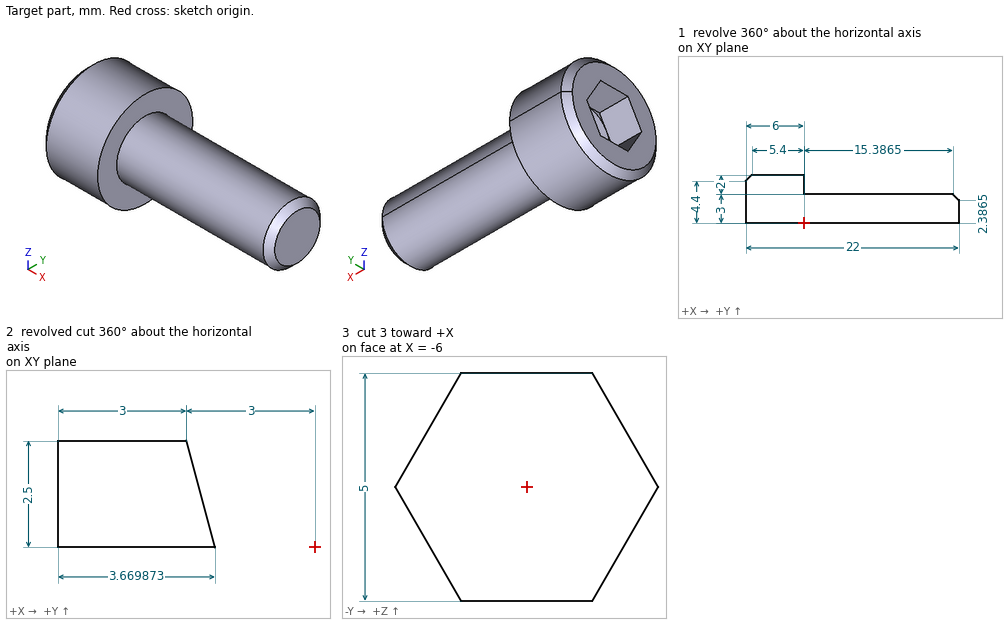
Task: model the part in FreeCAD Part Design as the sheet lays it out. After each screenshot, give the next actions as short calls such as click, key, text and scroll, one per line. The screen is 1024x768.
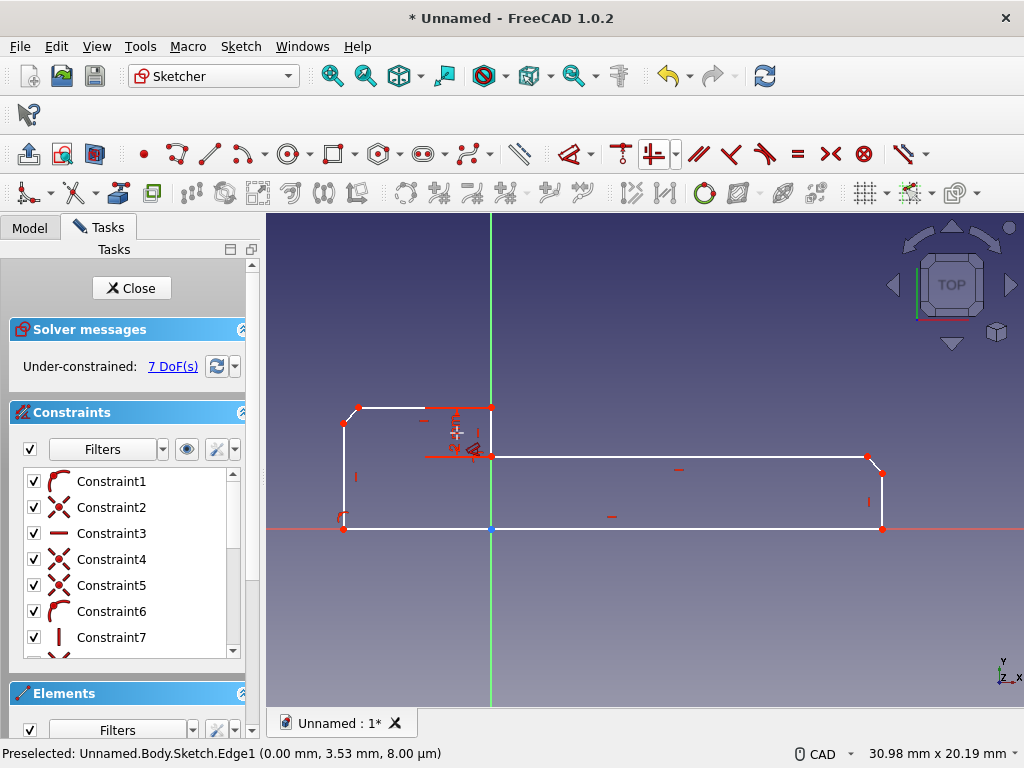
click(505, 529)
click(601, 563)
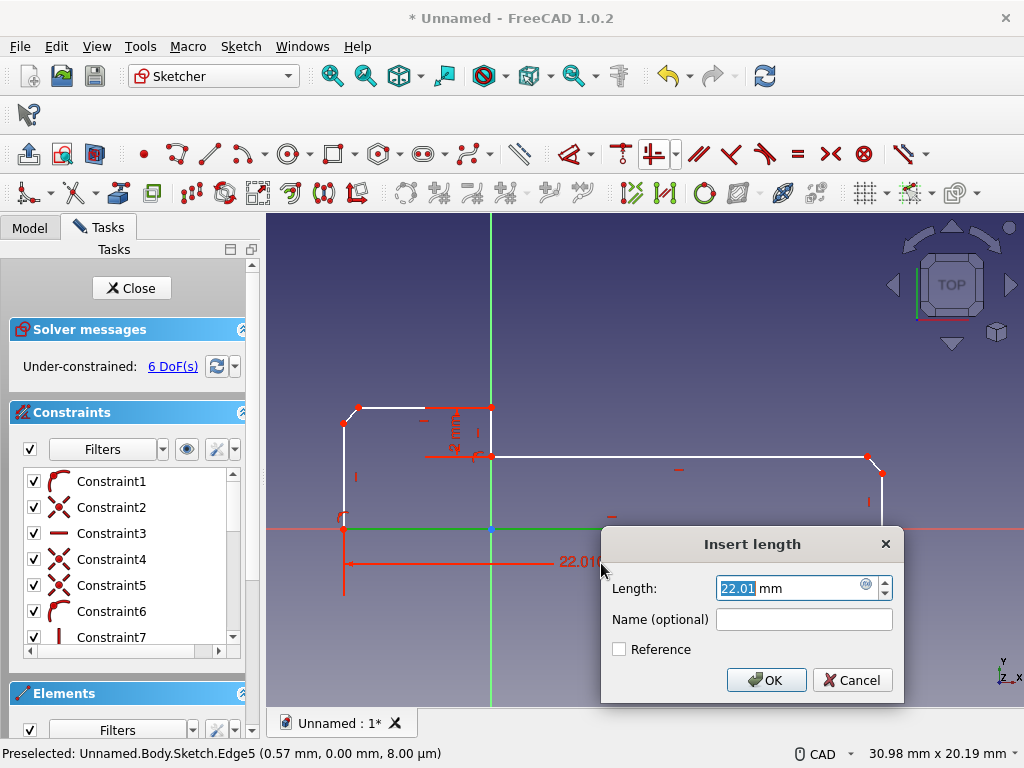
text(22)
key(Return)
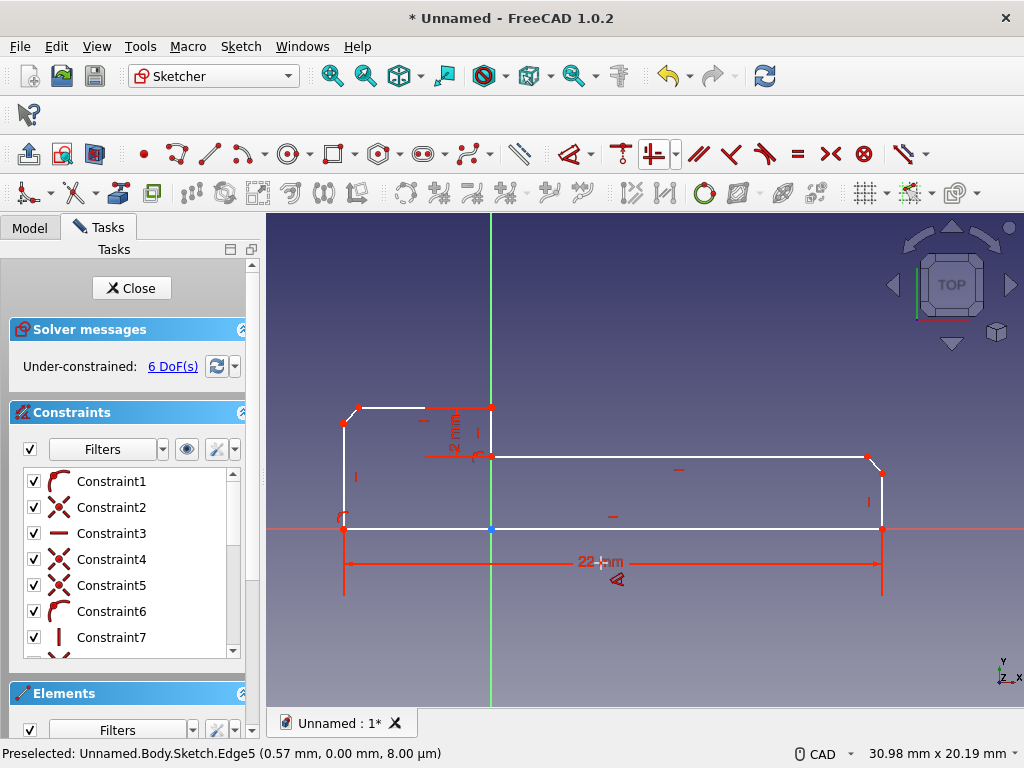
click(491, 457)
click(457, 493)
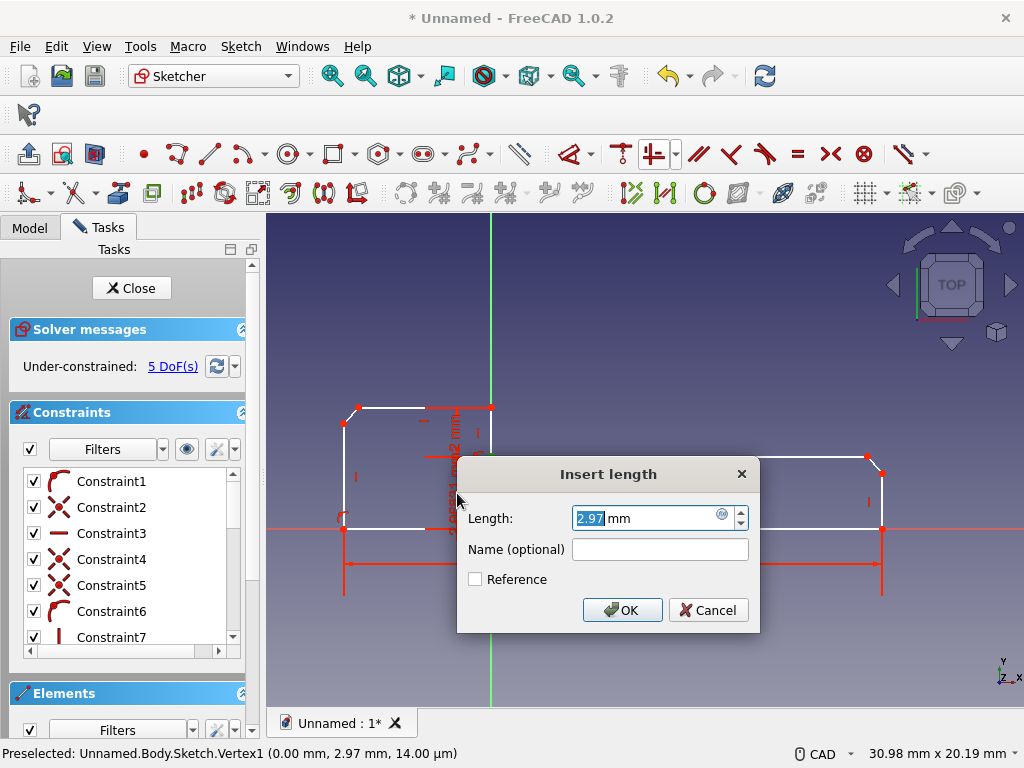
text(3)
key(Return)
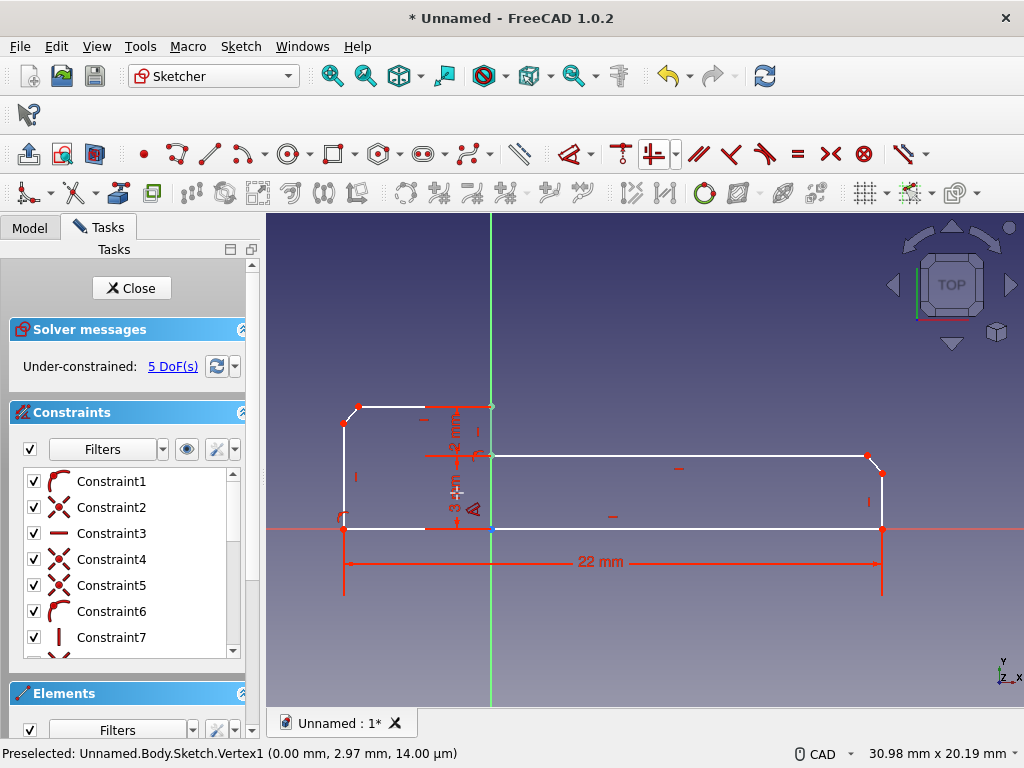
click(344, 424)
click(418, 563)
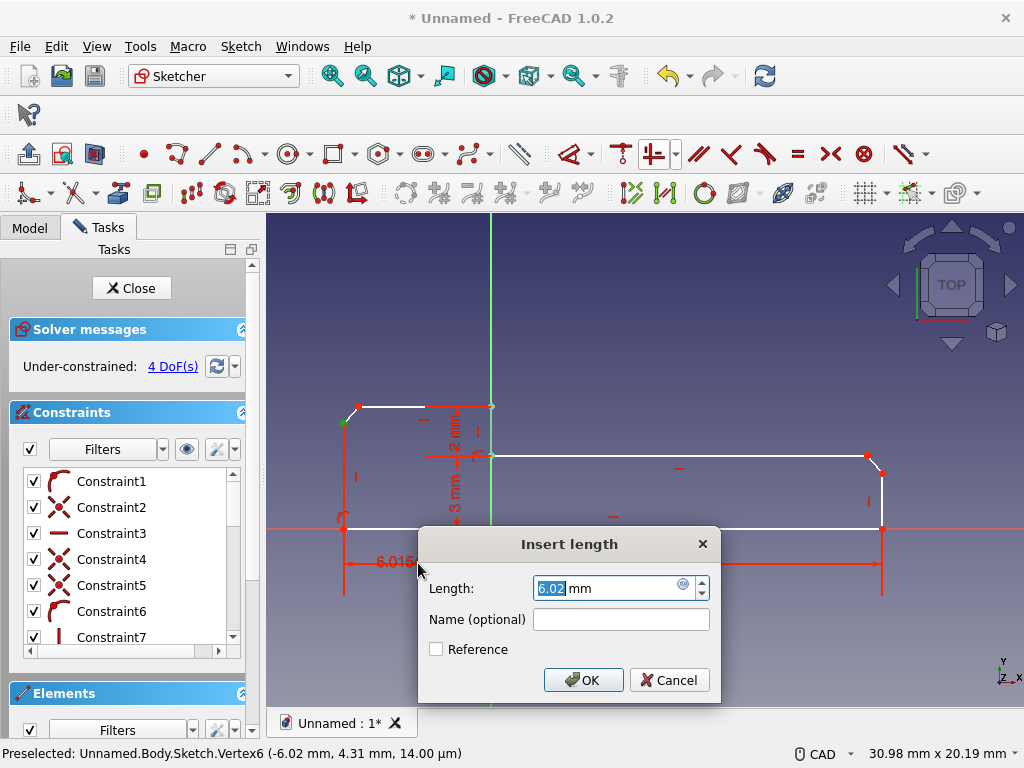
text(6)
key(Return)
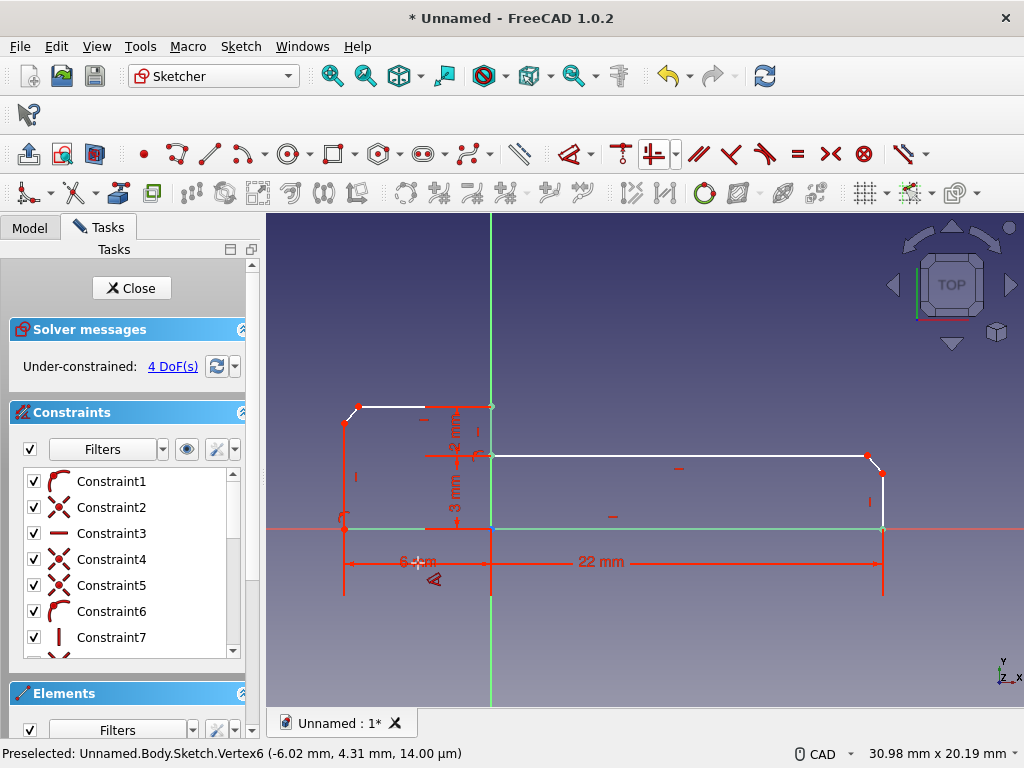
click(451, 407)
click(425, 373)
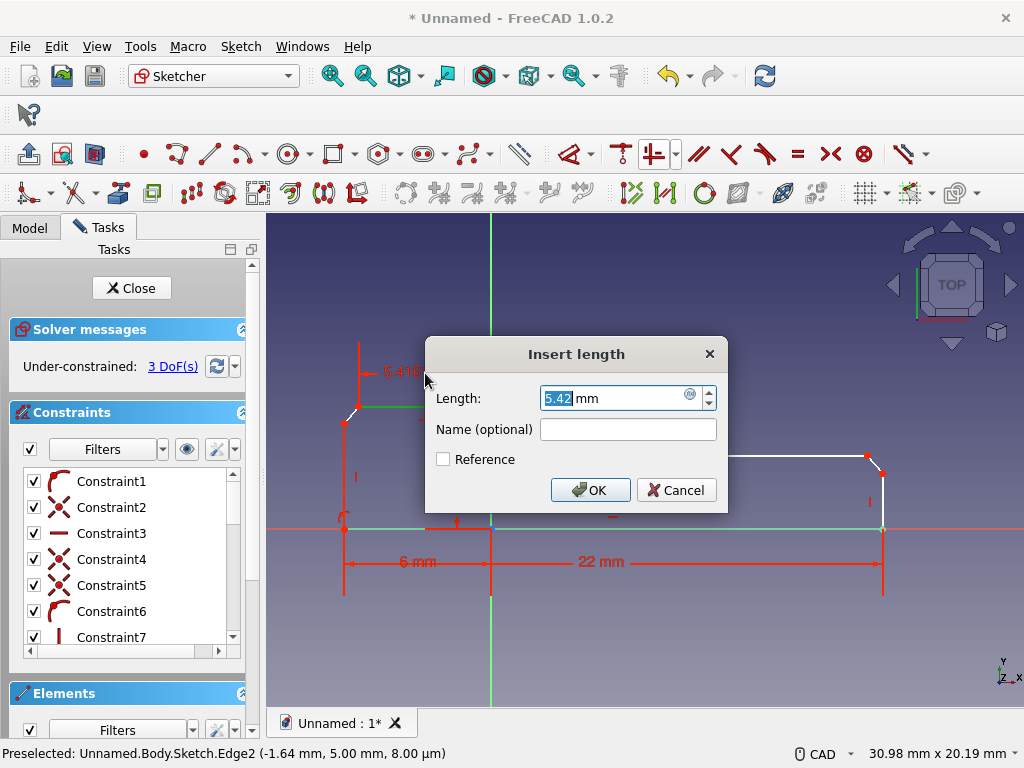
text(5.4)
key(Return)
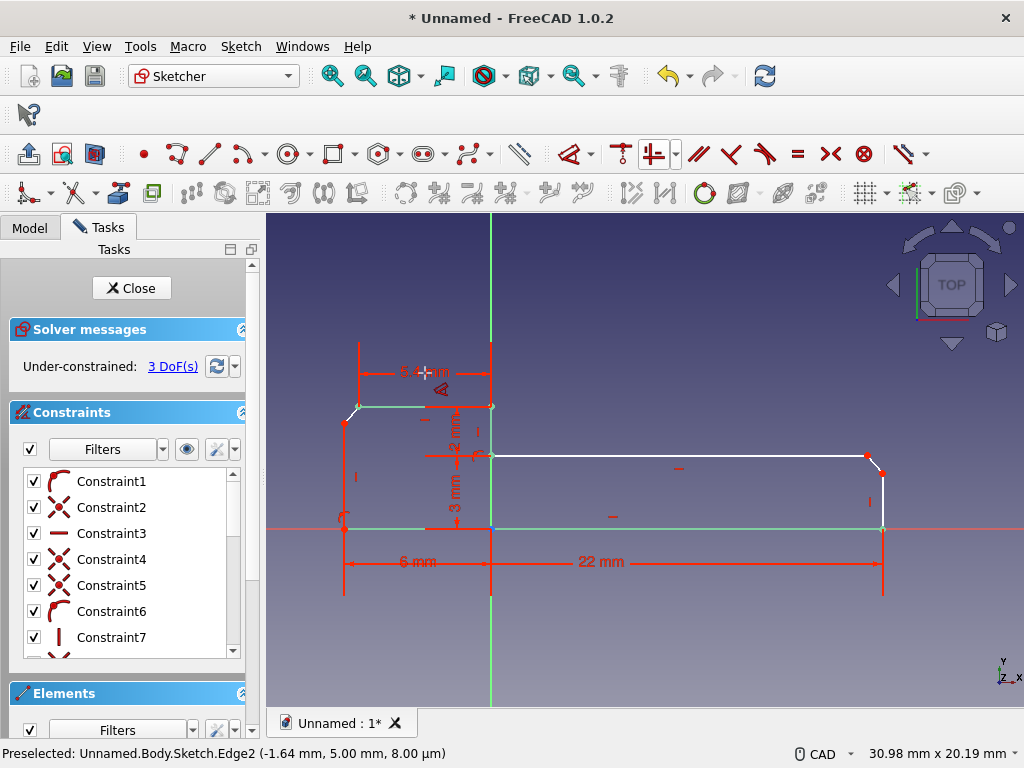
click(344, 456)
click(310, 477)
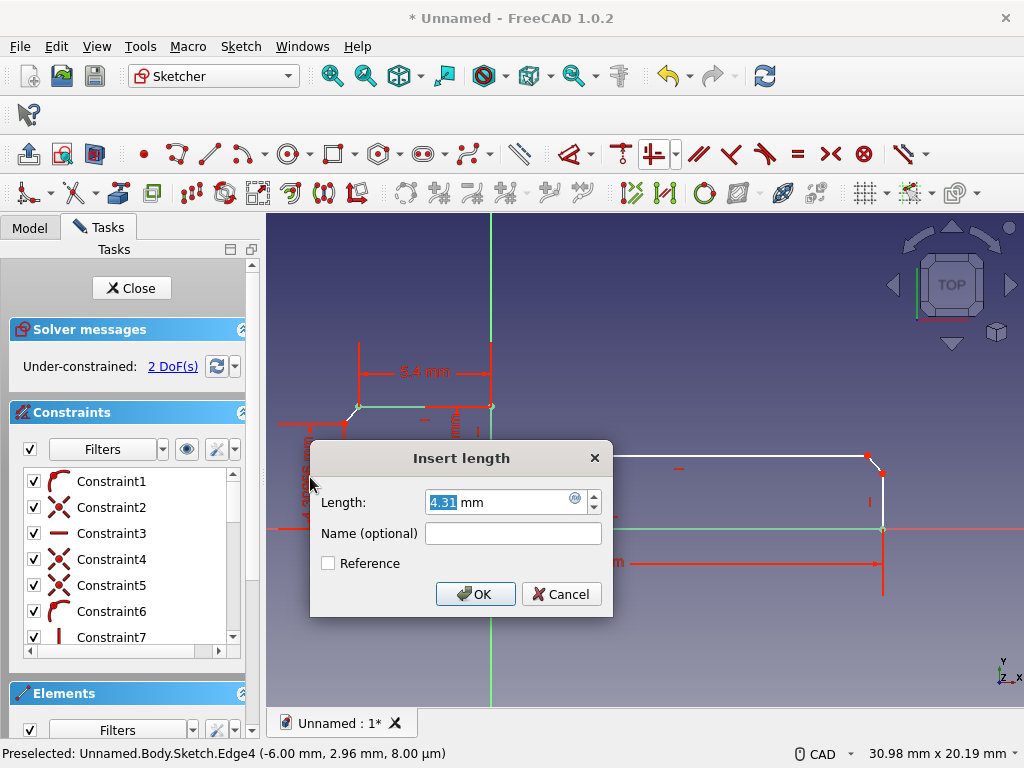
text(4.4)
key(Return)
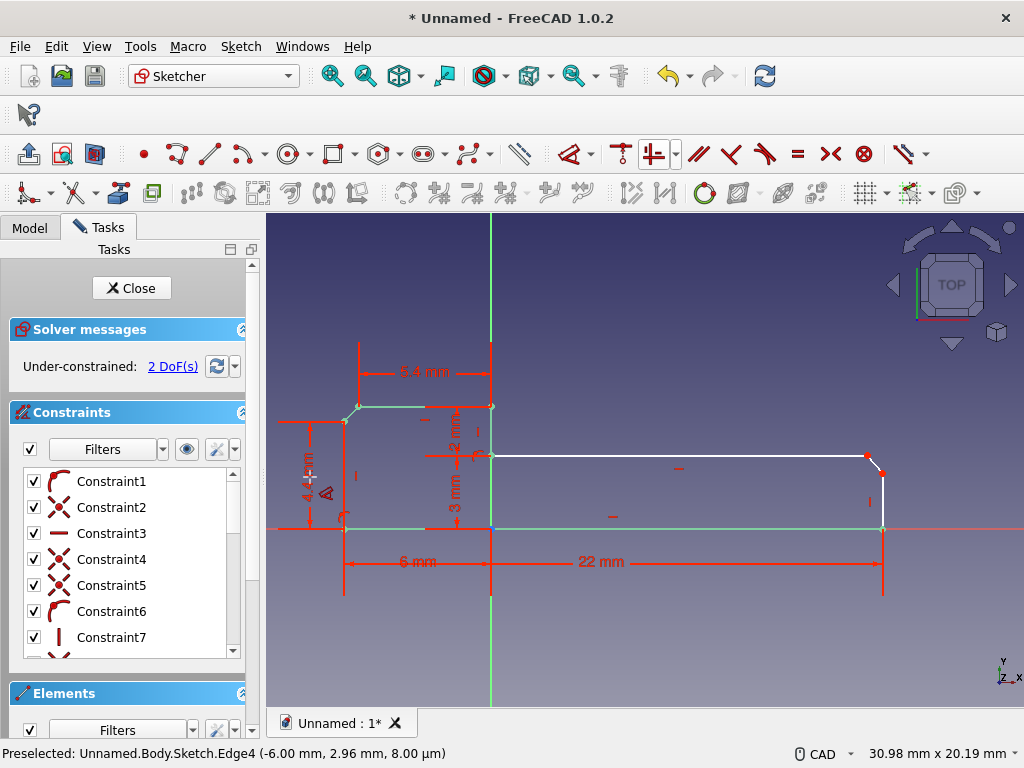
scroll(501, 443, down, 2)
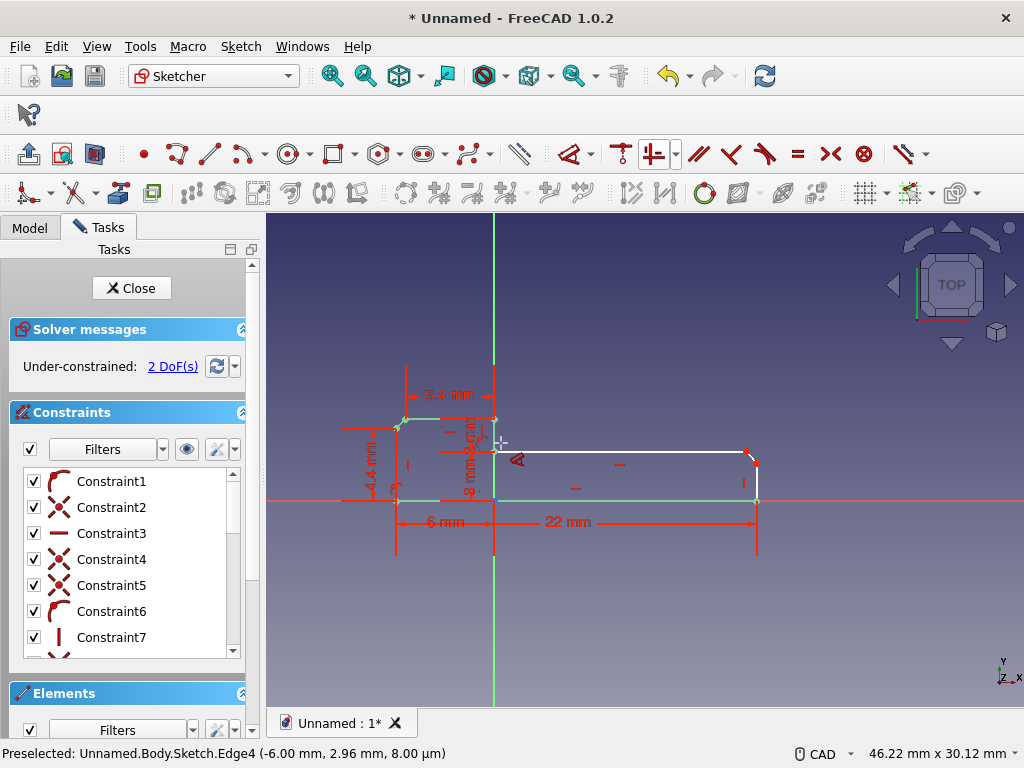
click(757, 490)
click(791, 482)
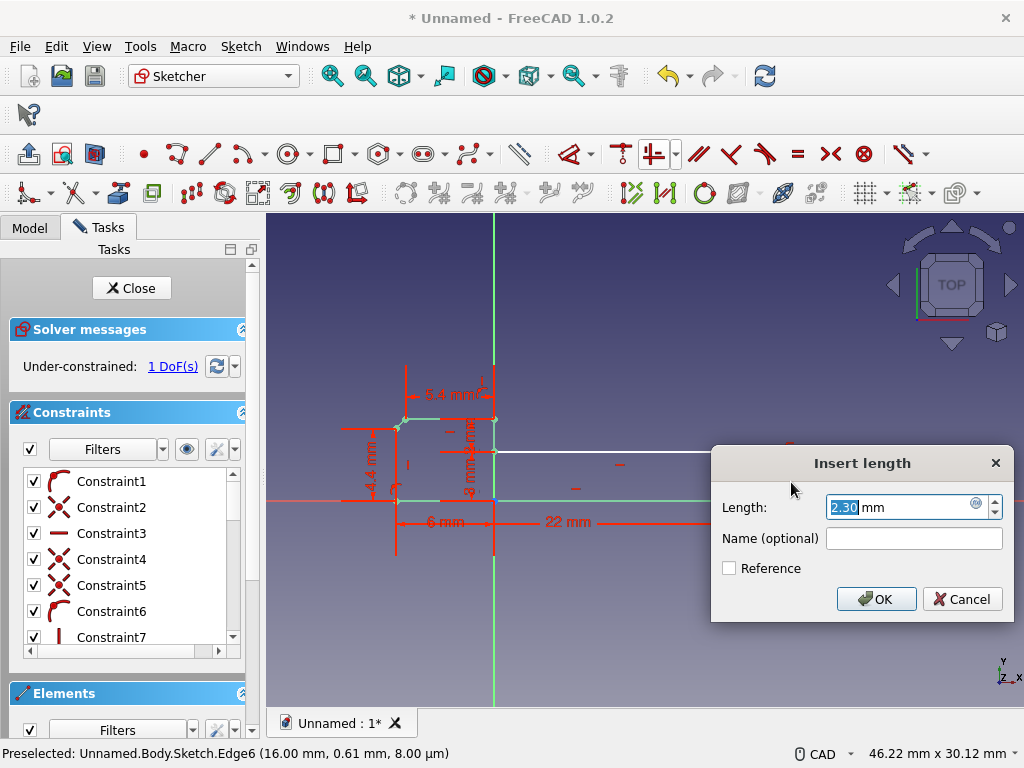
text(2.3865)
key(Return)